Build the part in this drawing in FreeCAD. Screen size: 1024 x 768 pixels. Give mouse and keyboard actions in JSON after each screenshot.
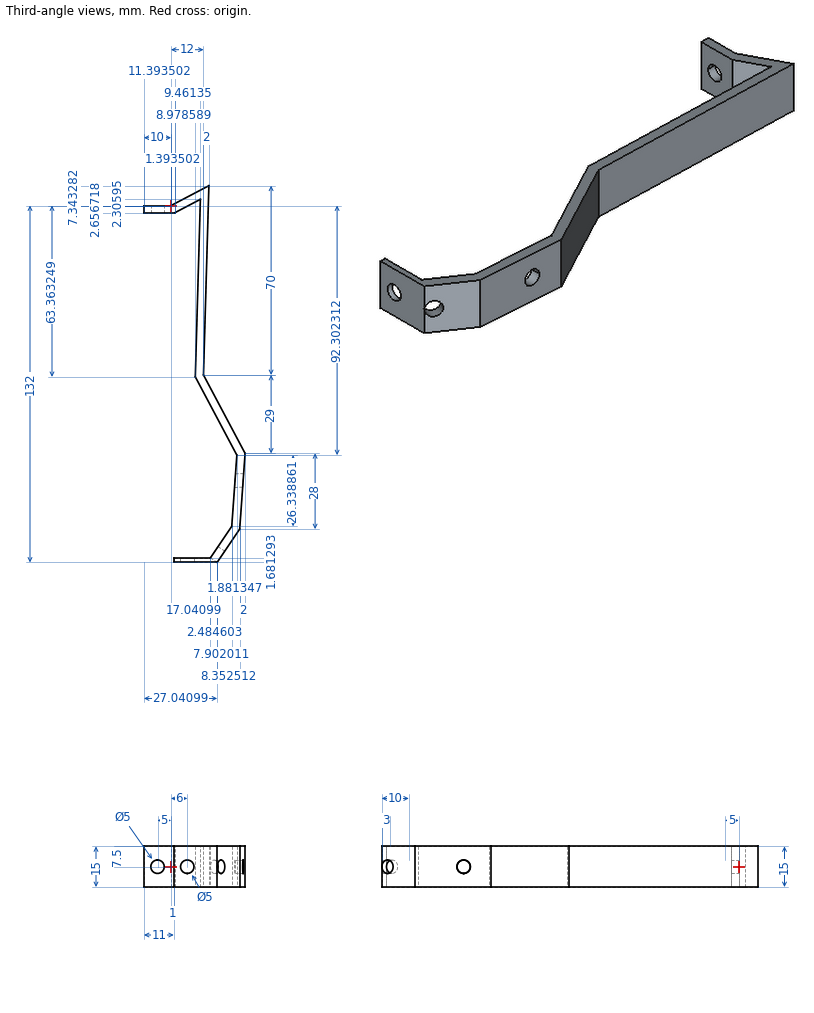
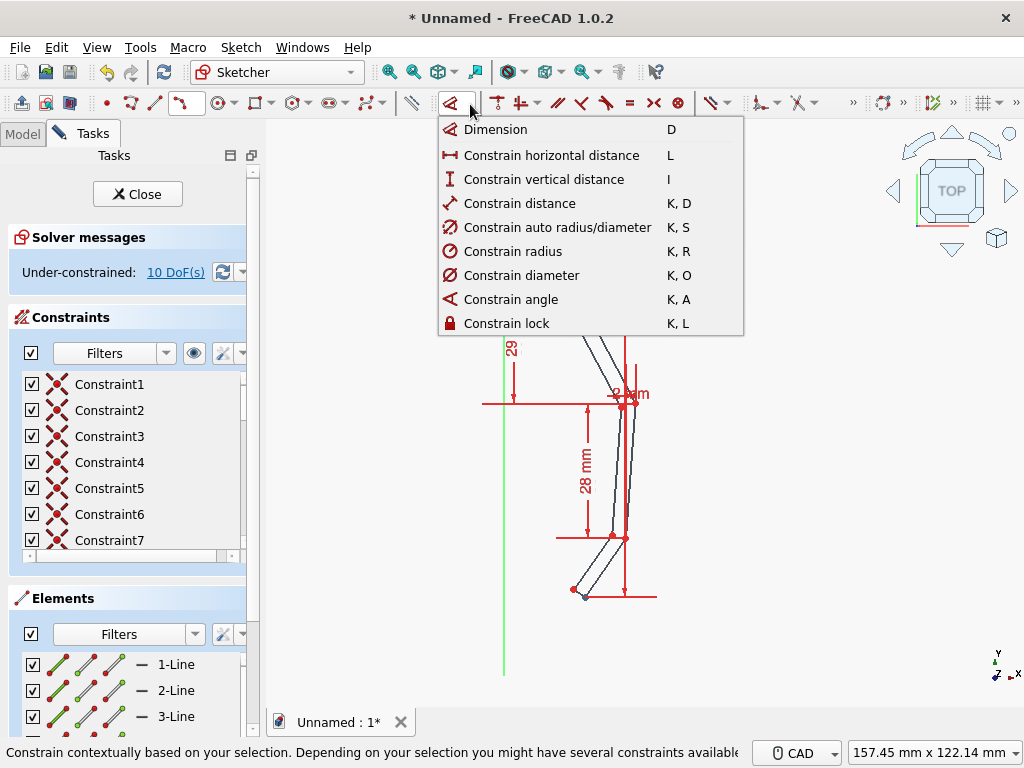
{"action": "left_click", "coordinate": [591, 155]}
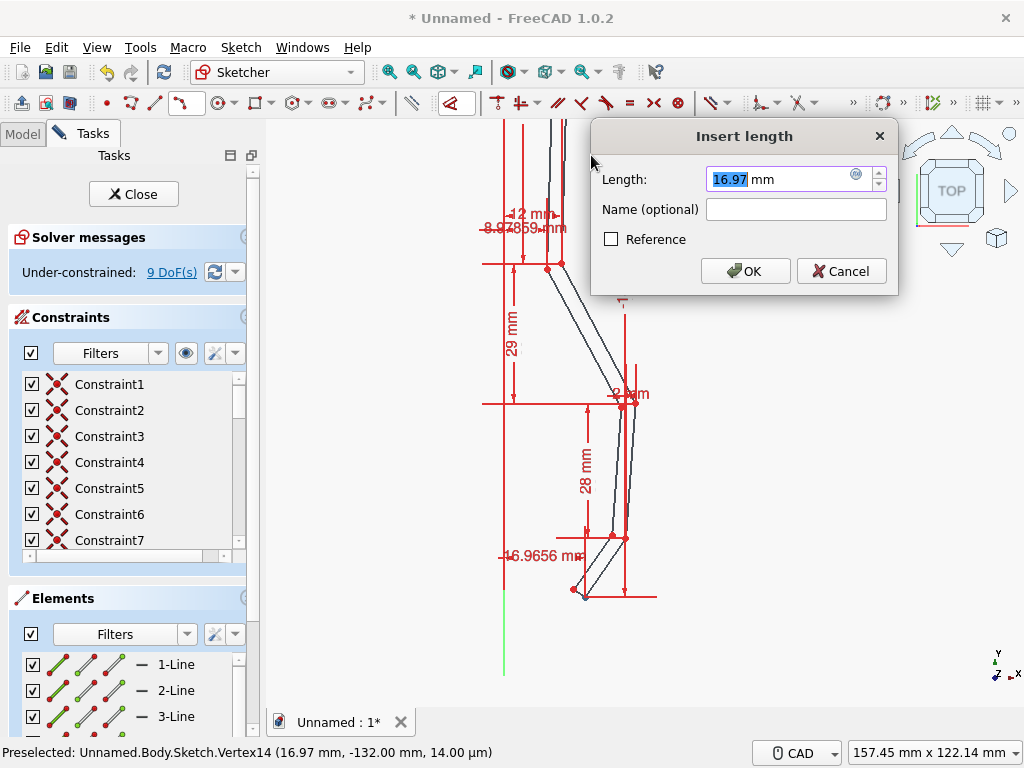
{"action": "type", "text": "17.04099"}
{"action": "key", "text": "Return"}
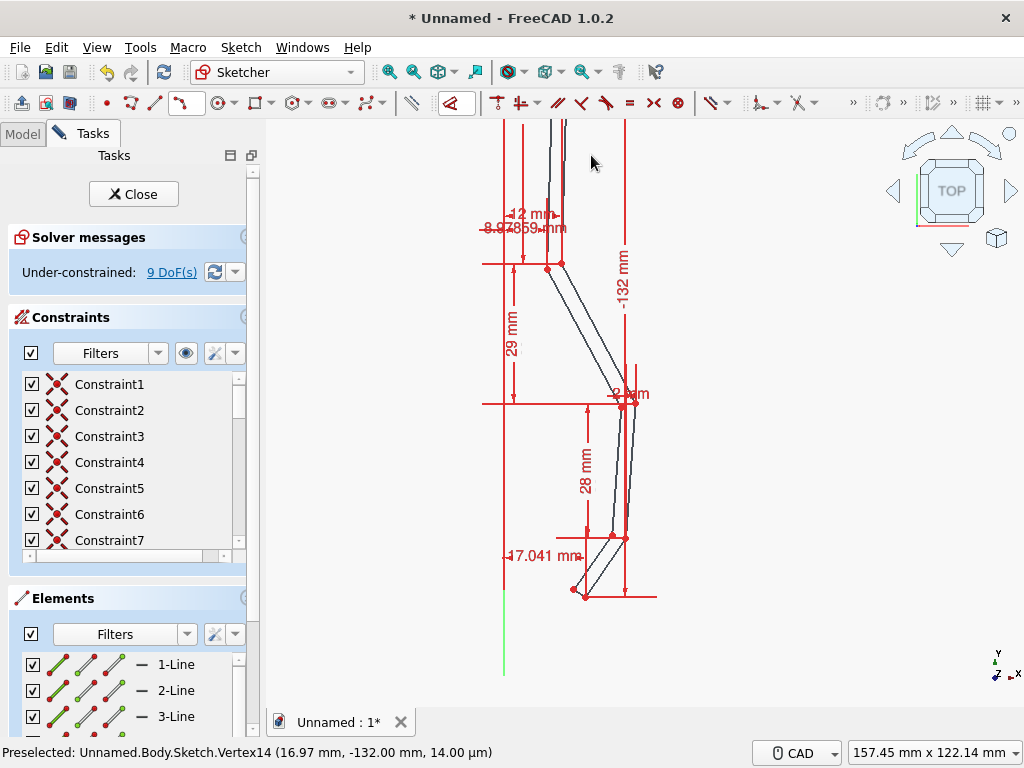
{"action": "scroll", "coordinate": [585, 597], "scroll_direction": "down", "scroll_amount": 3}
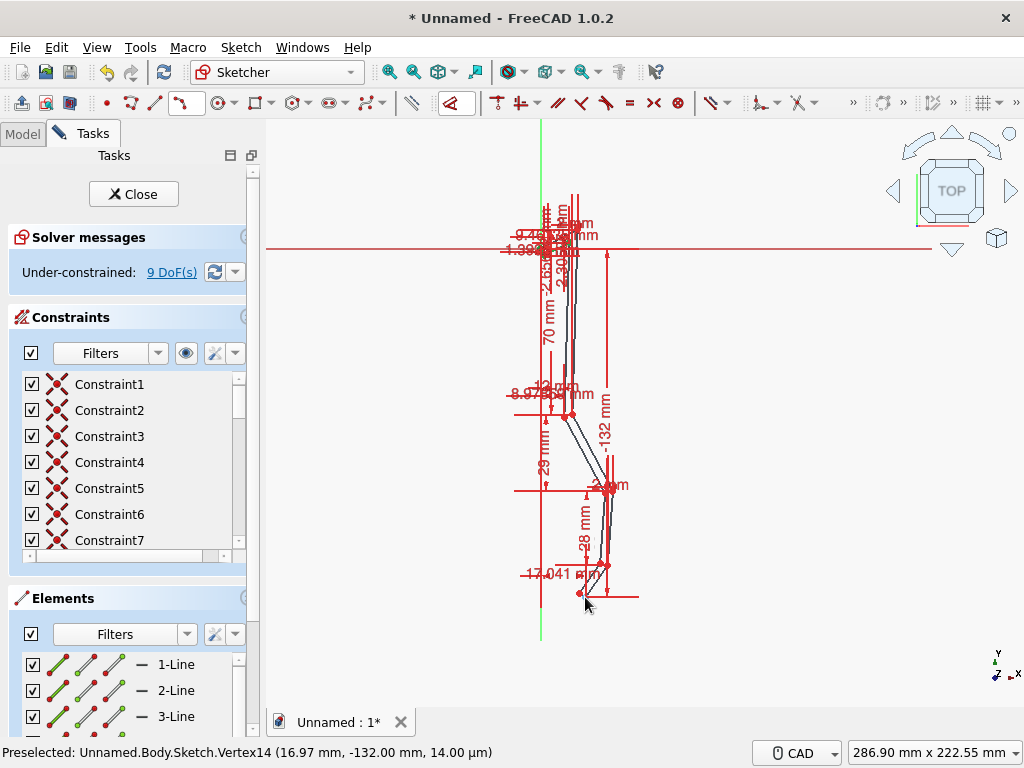
{"action": "scroll", "coordinate": [578, 230], "scroll_direction": "up", "scroll_amount": 4}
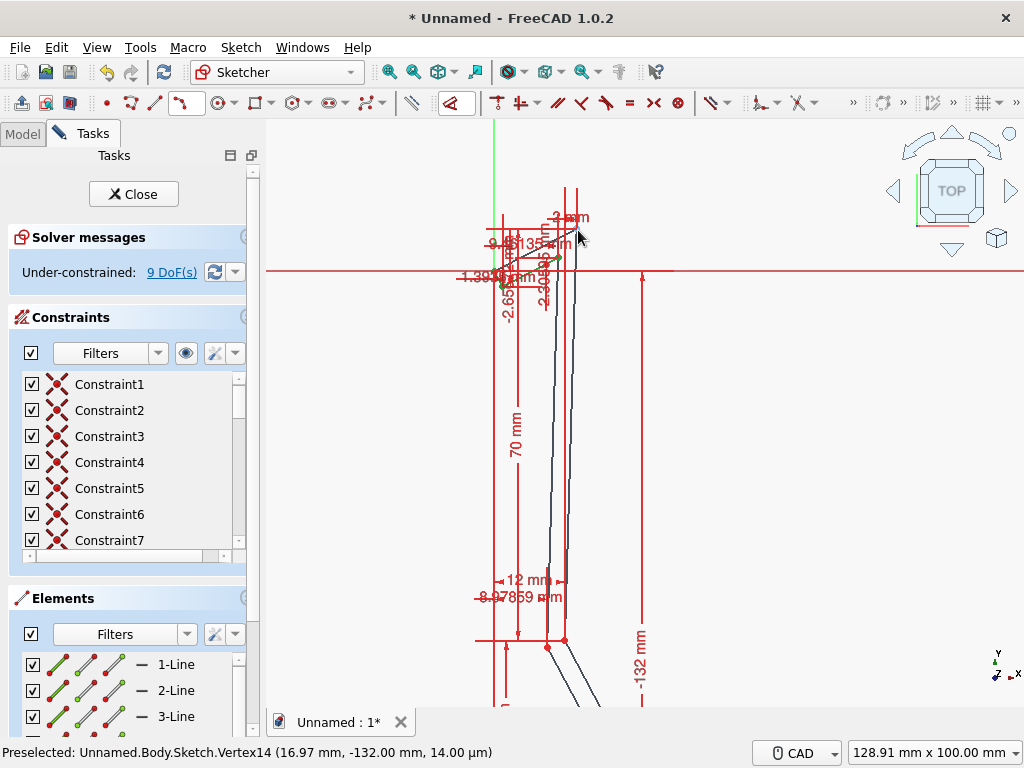
{"action": "left_click", "coordinate": [577, 229]}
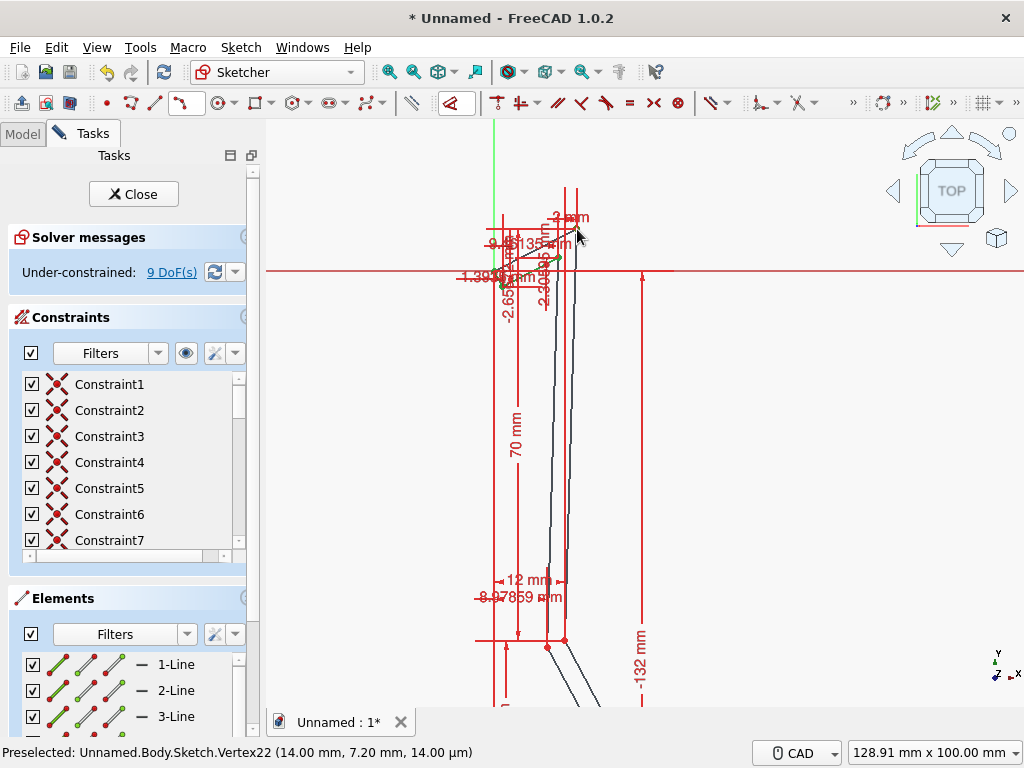
{"action": "key", "text": "i"}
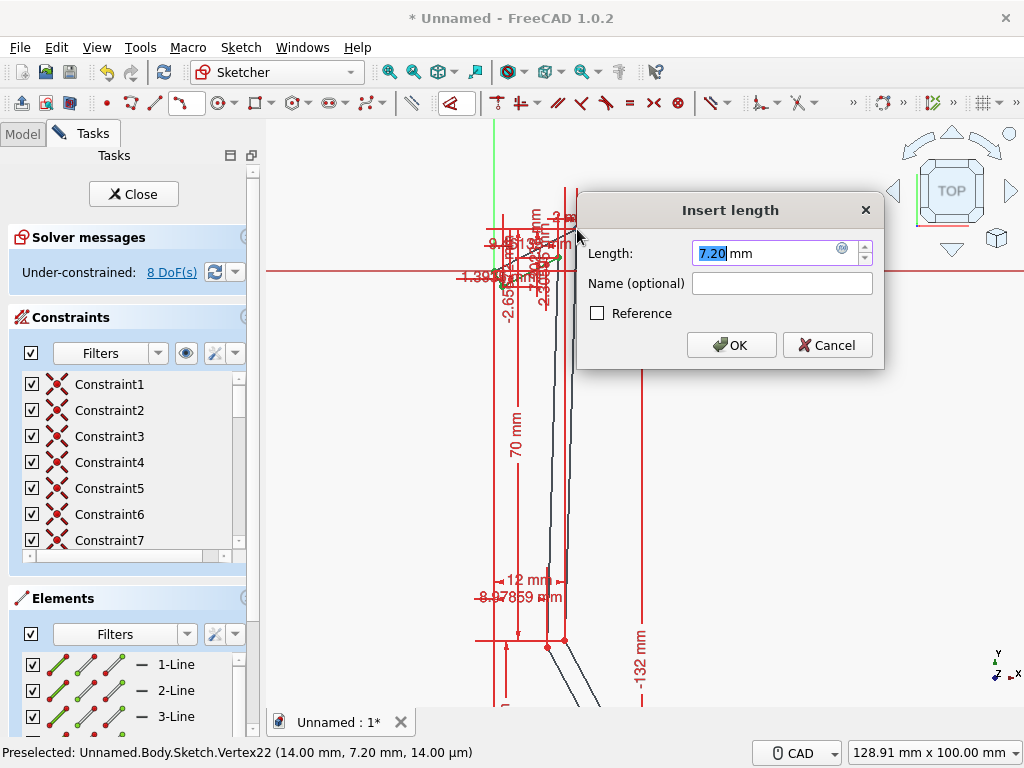
{"action": "type", "text": "7.343282"}
{"action": "key", "text": "Return"}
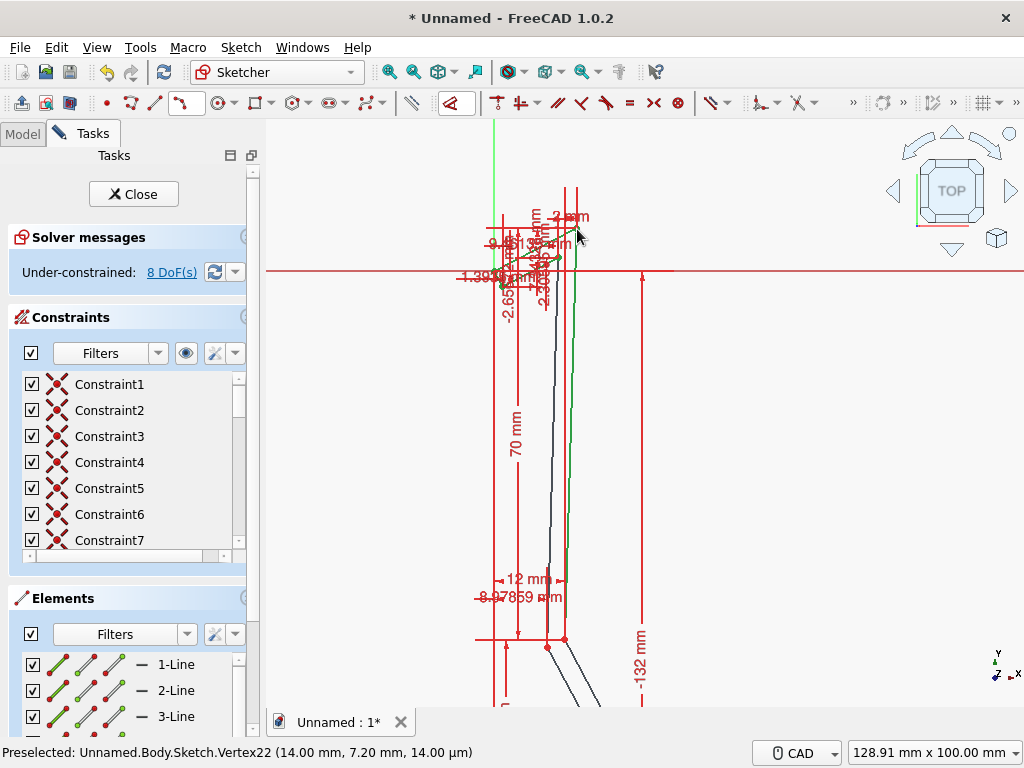
{"action": "scroll", "coordinate": [578, 230], "scroll_direction": "down", "scroll_amount": 4}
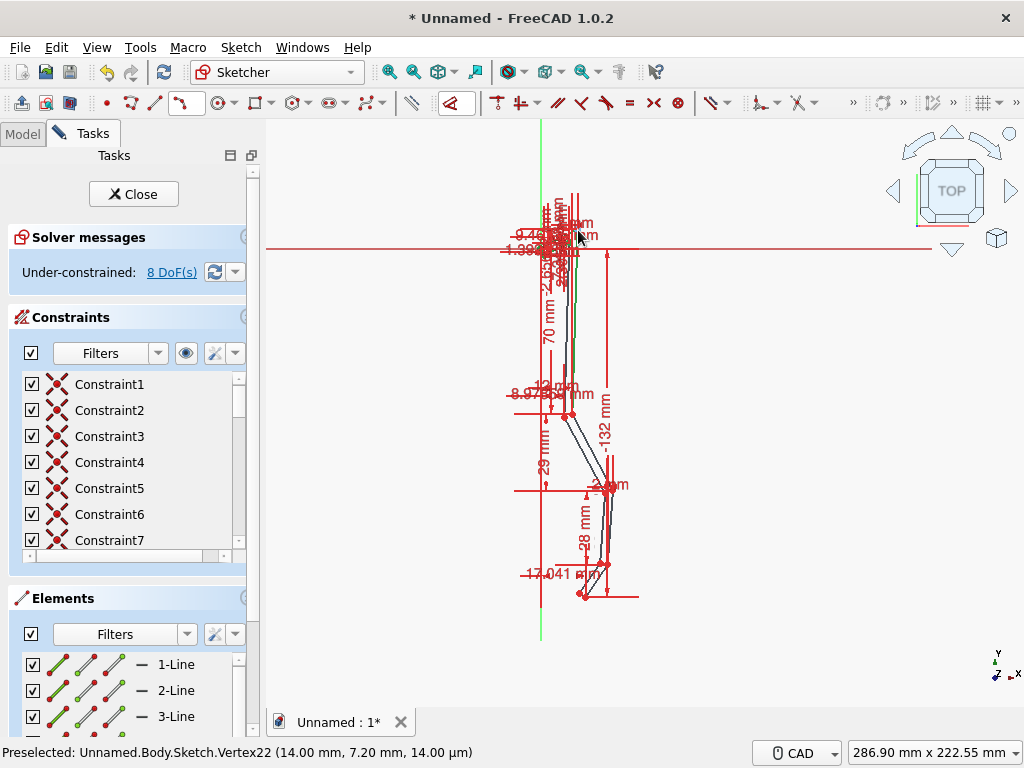
{"action": "scroll", "coordinate": [604, 515], "scroll_direction": "up", "scroll_amount": 11}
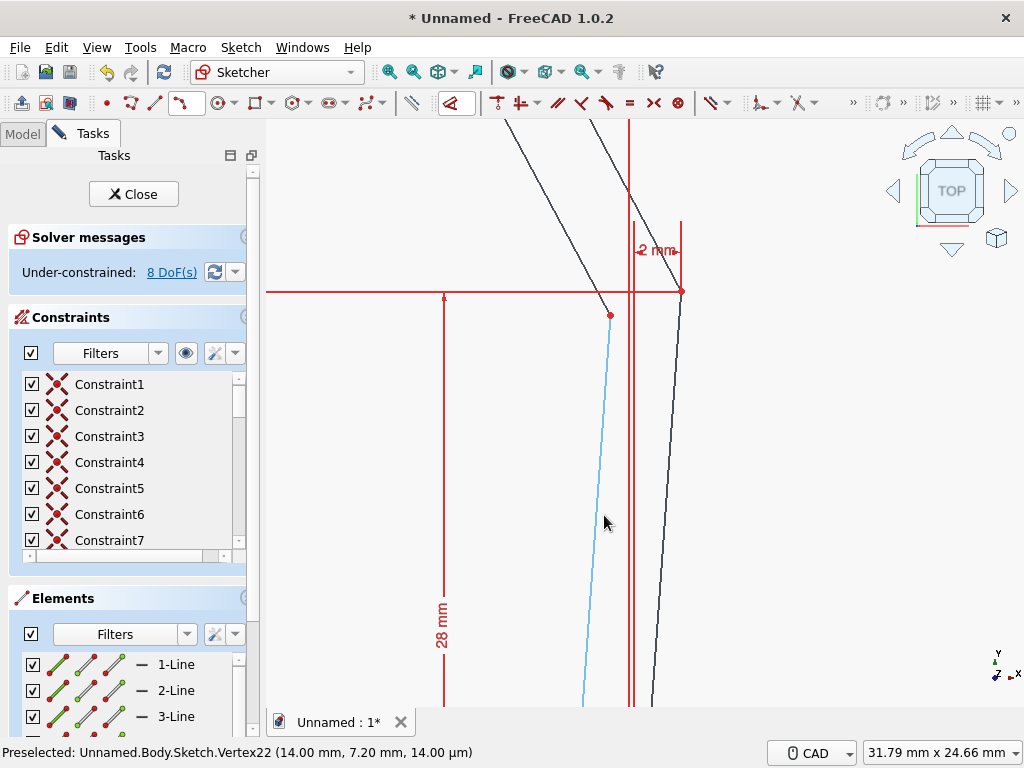
{"action": "left_click", "coordinate": [597, 505]}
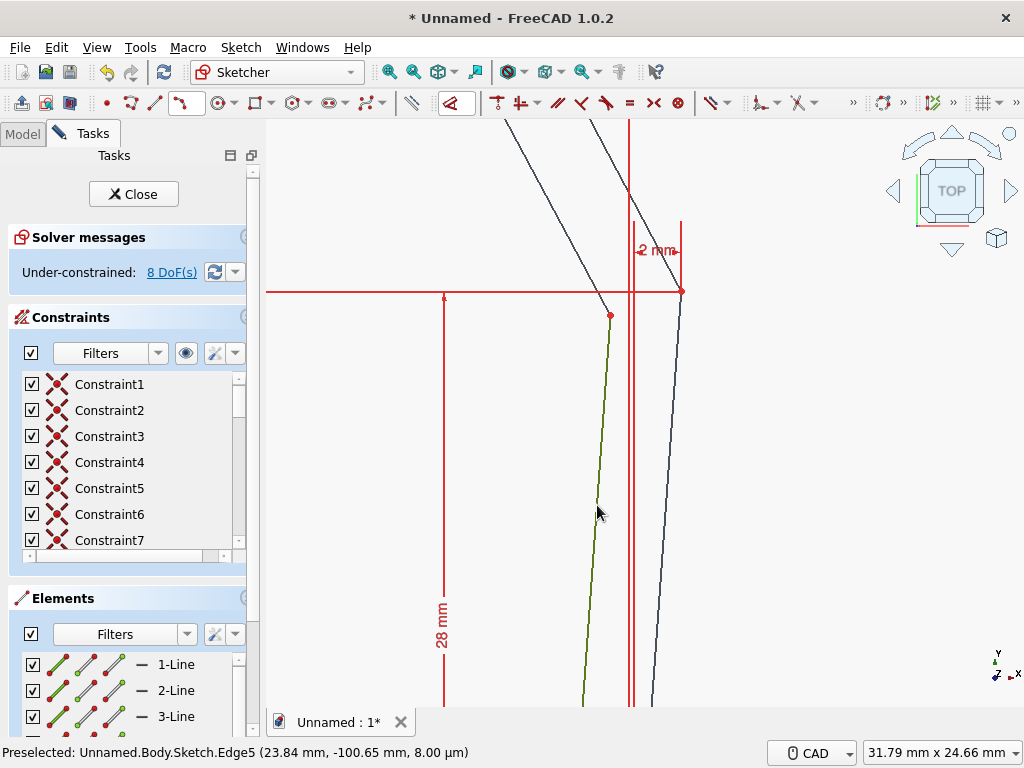
{"action": "left_click", "coordinate": [470, 104]}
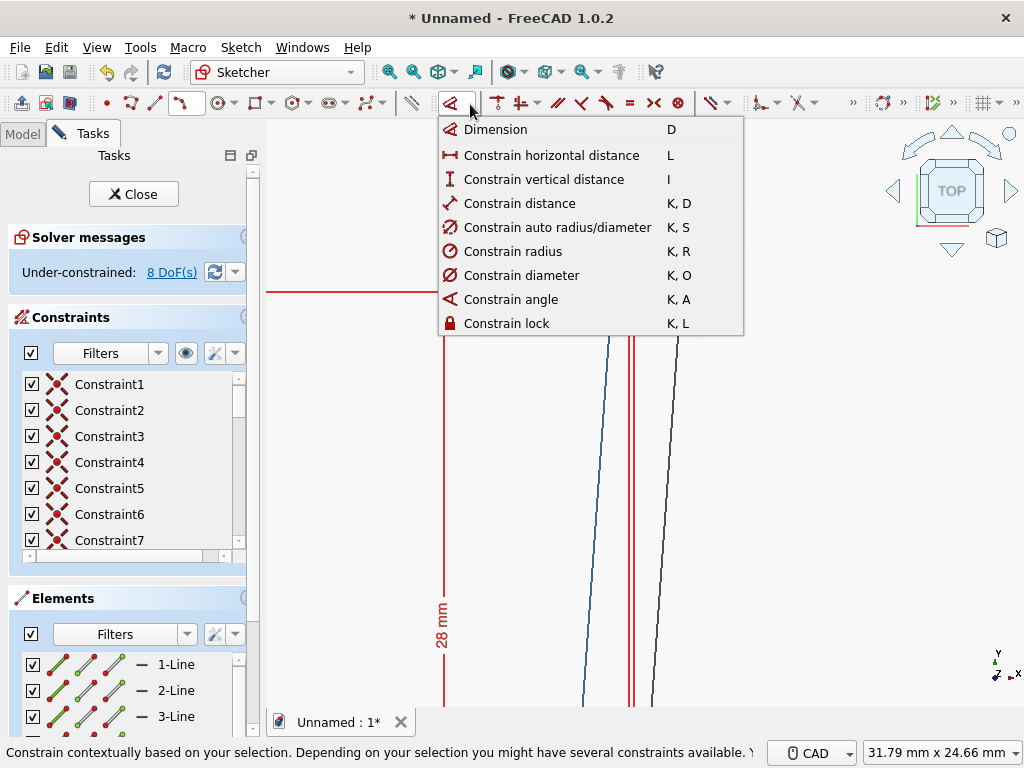
{"action": "left_click", "coordinate": [591, 155]}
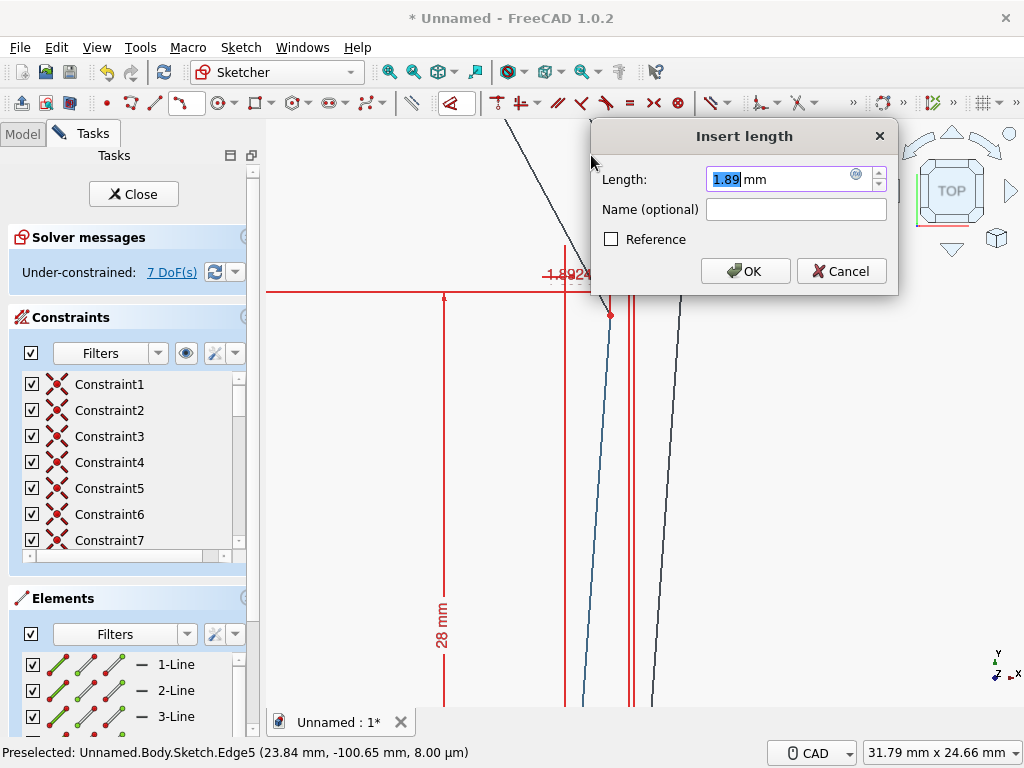
{"action": "type", "text": "1.881347"}
{"action": "key", "text": "Return"}